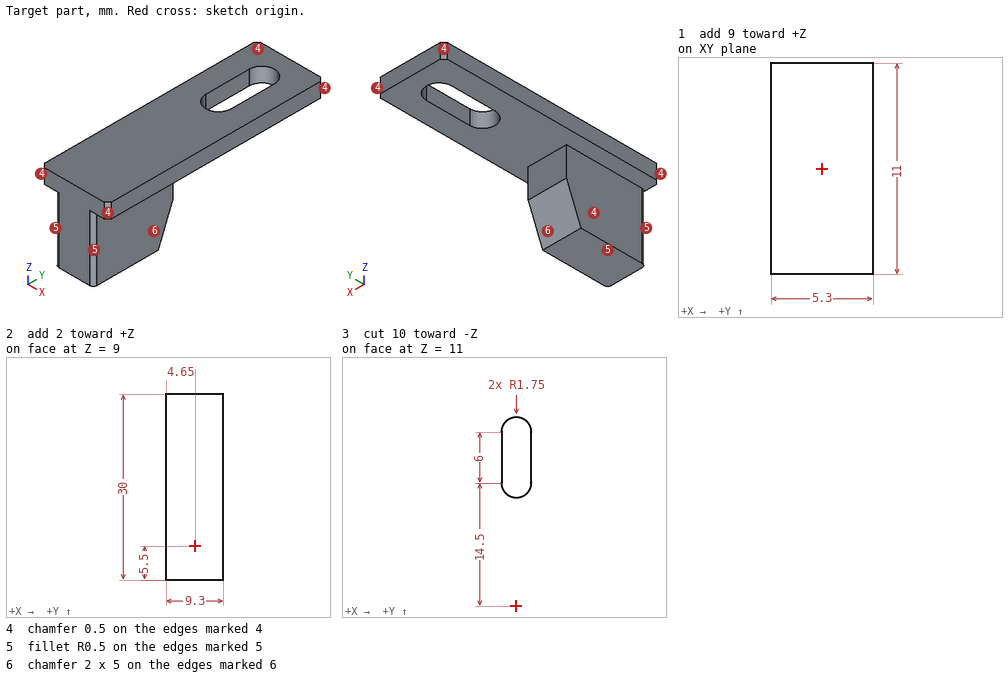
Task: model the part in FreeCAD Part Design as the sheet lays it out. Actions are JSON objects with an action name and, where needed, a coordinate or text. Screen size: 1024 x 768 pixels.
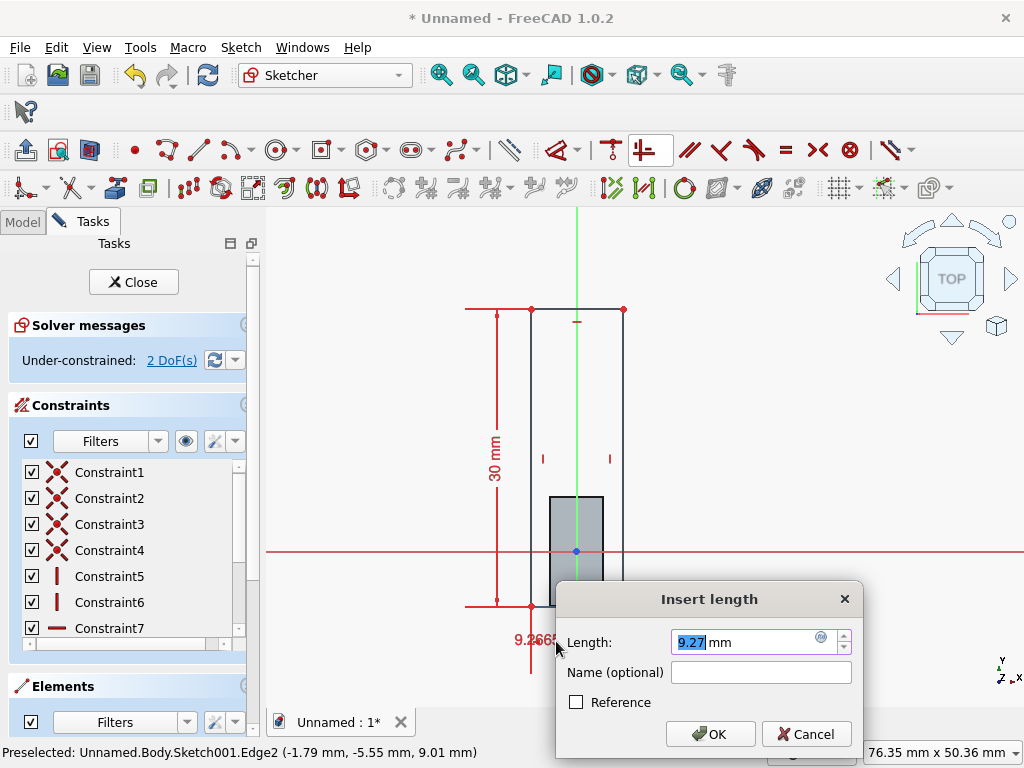
{"action": "type", "text": "9.3"}
{"action": "key", "text": "Return"}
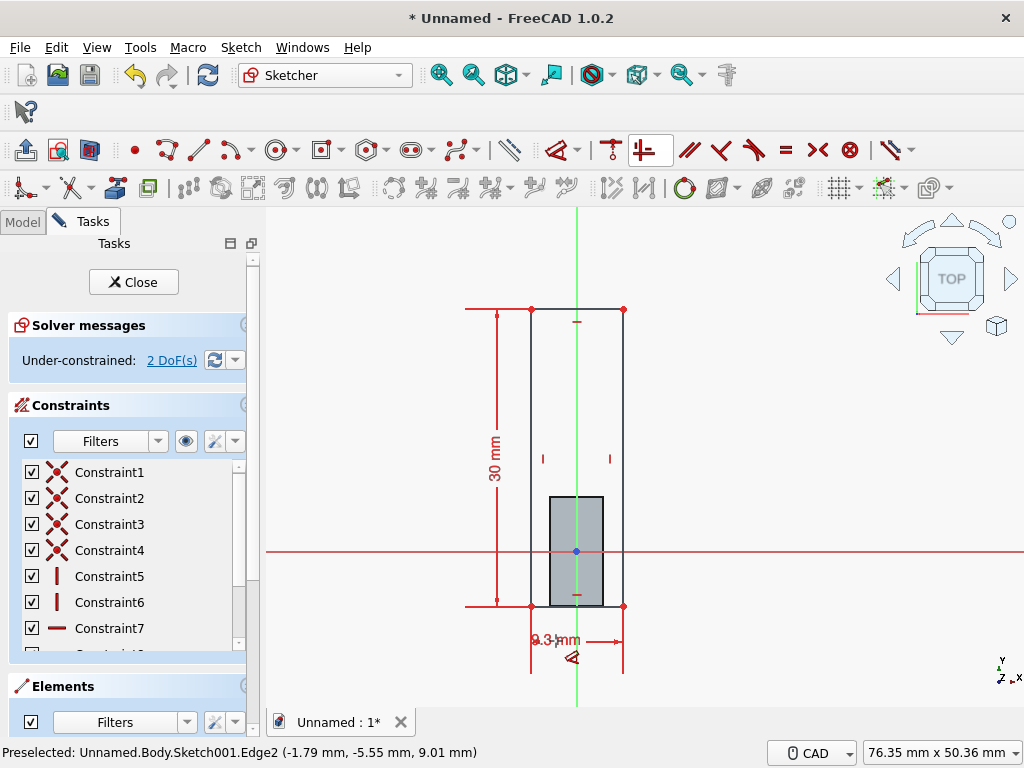
{"action": "left_click", "coordinate": [531, 607]}
{"action": "left_click", "coordinate": [497, 579]}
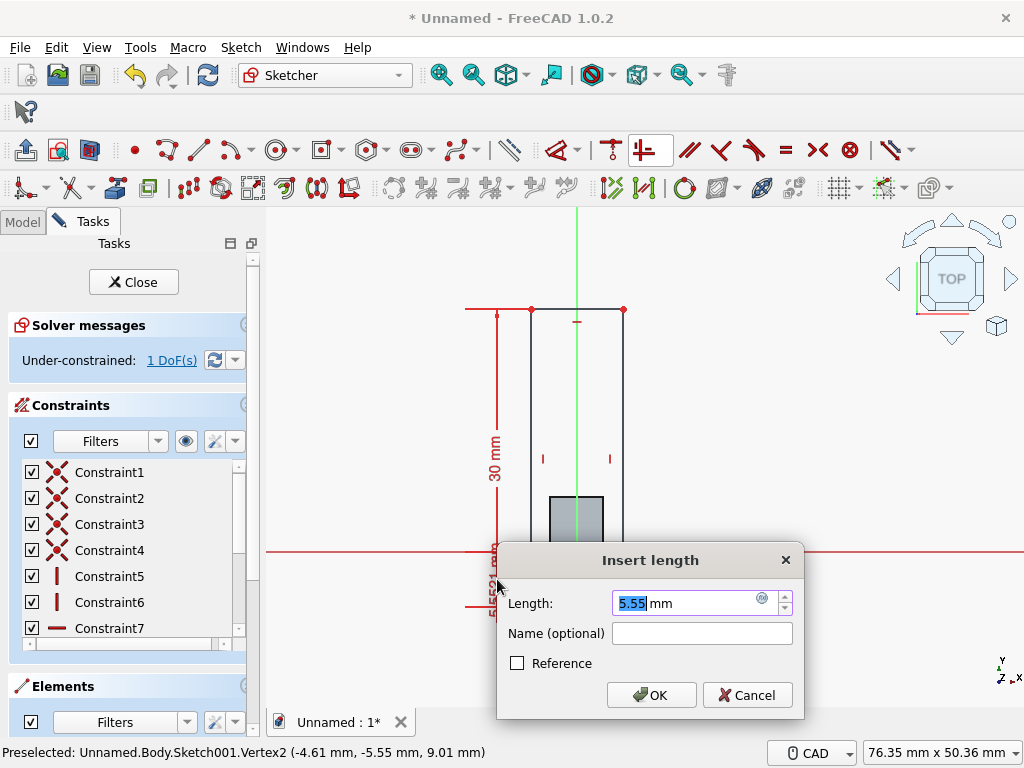
{"action": "type", "text": "5.5"}
{"action": "key", "text": "Return"}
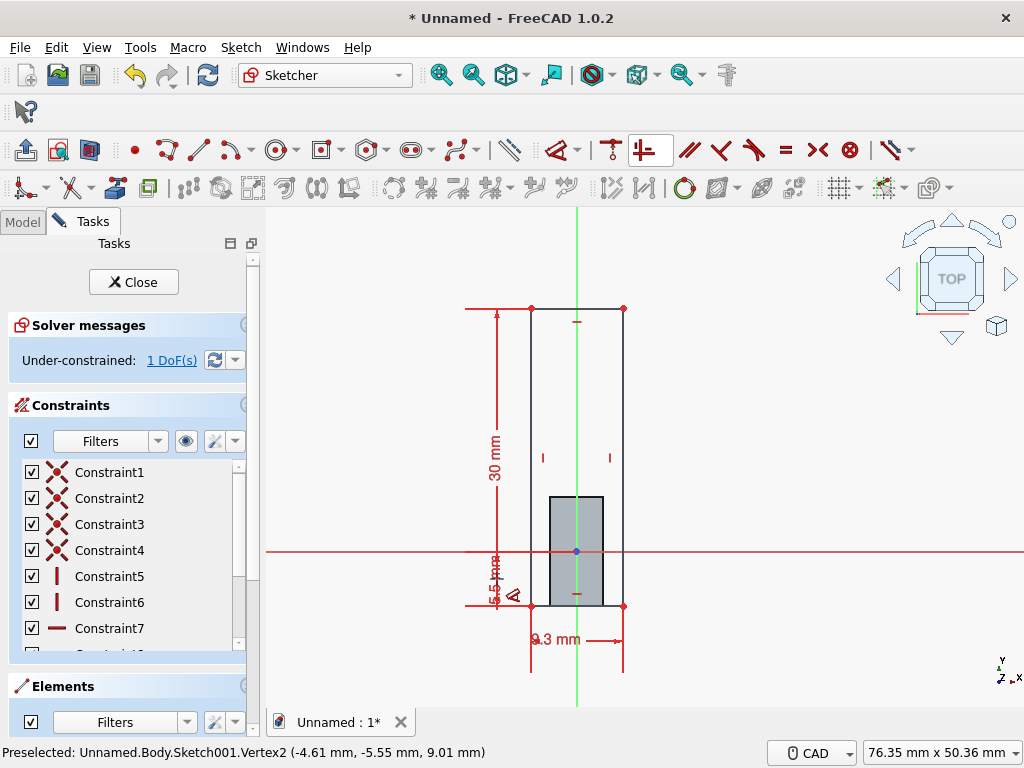
{"action": "left_click", "coordinate": [531, 309]}
{"action": "left_click", "coordinate": [554, 275]}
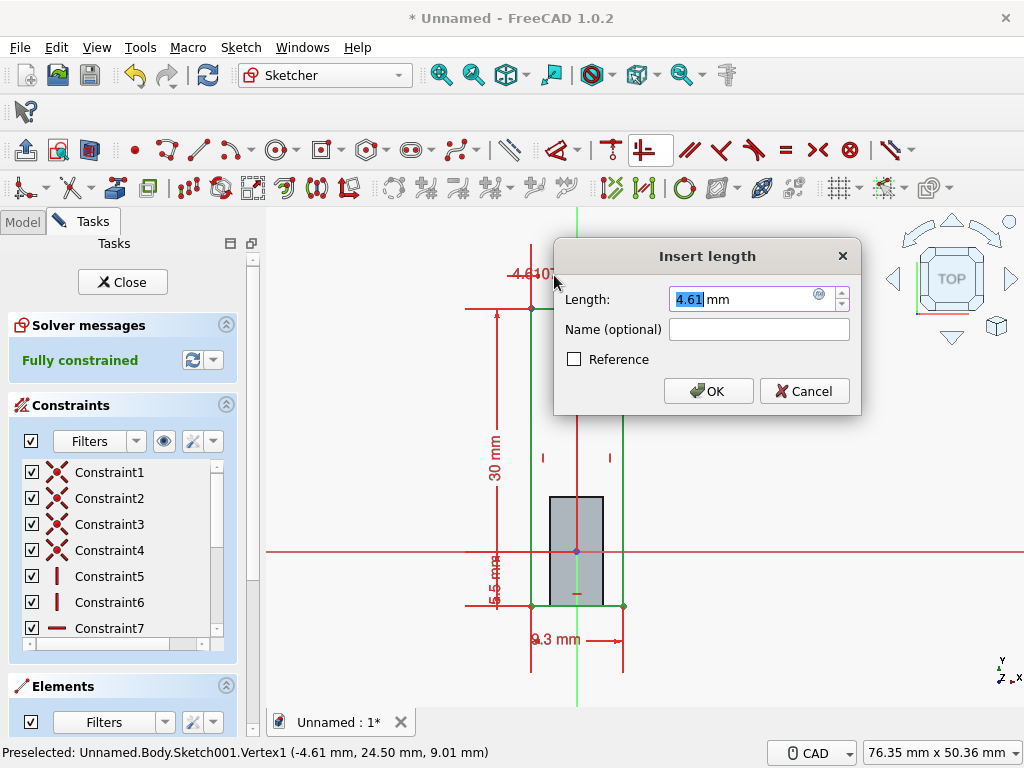
{"action": "type", "text": "4.65"}
{"action": "key", "text": "Return"}
{"action": "key", "text": "Escape"}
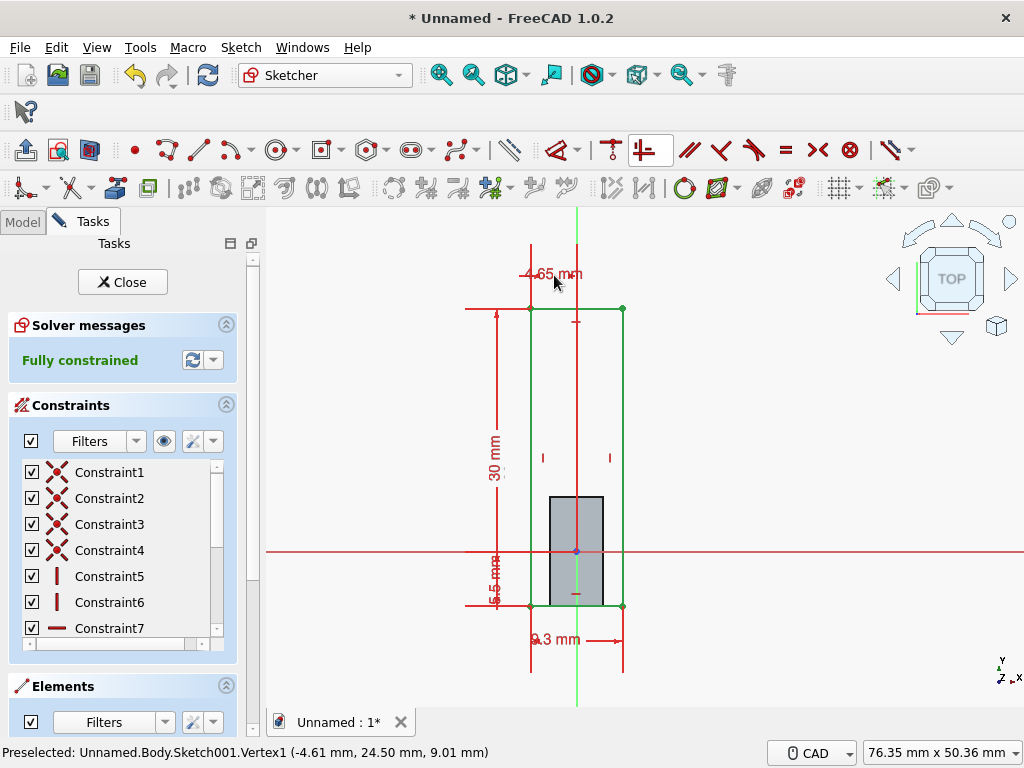
{"action": "left_click", "coordinate": [123, 282]}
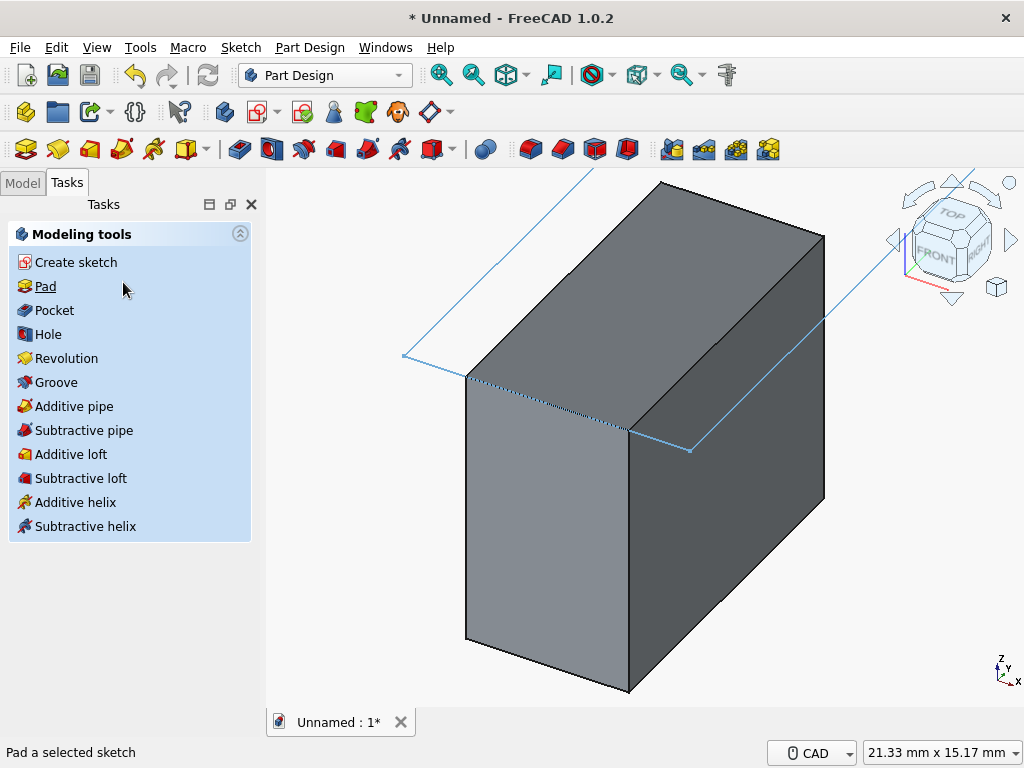
{"action": "left_click", "coordinate": [26, 150]}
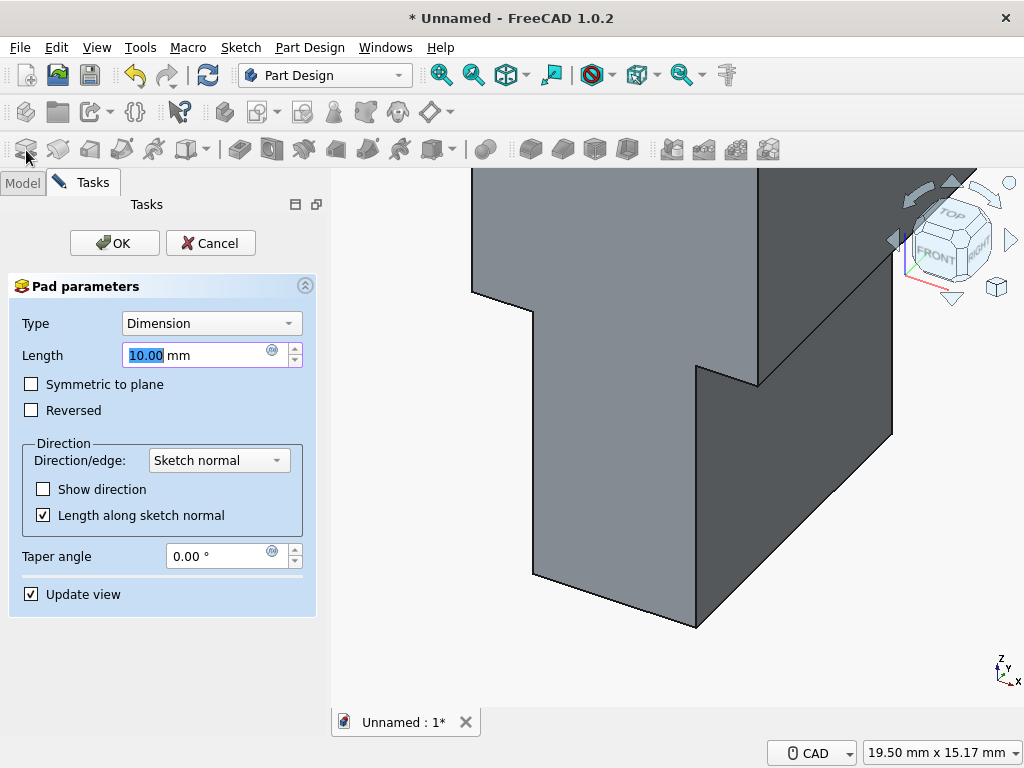
{"action": "type", "text": "2"}
{"action": "key", "text": "Tab"}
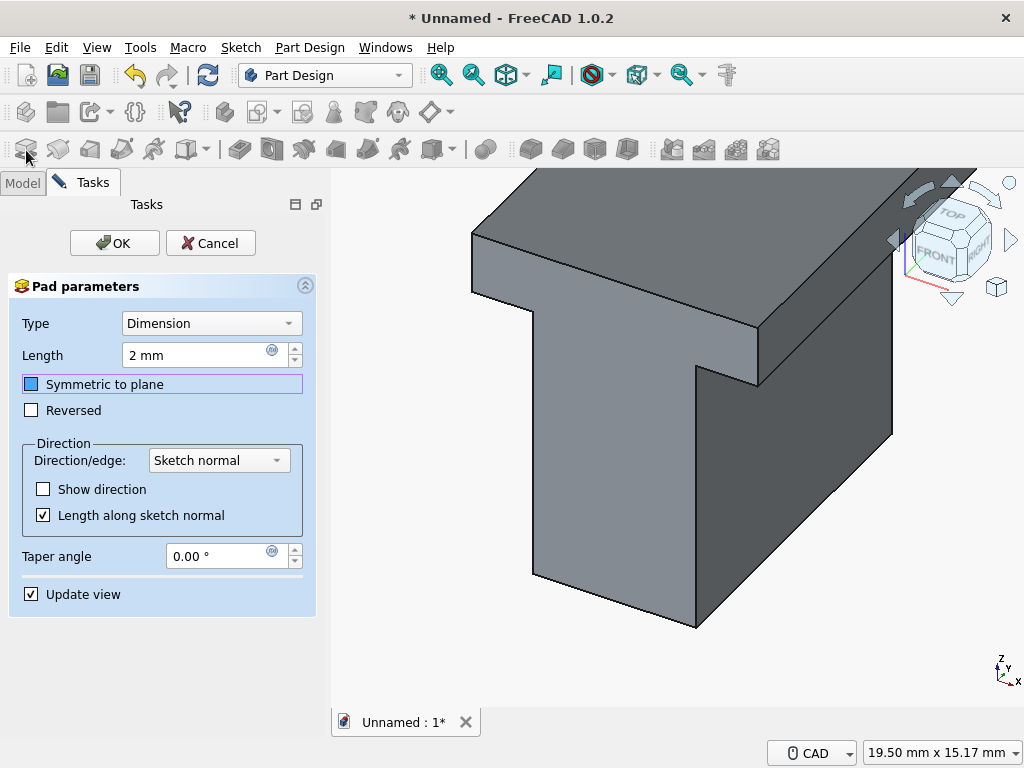
{"action": "left_click", "coordinate": [115, 243]}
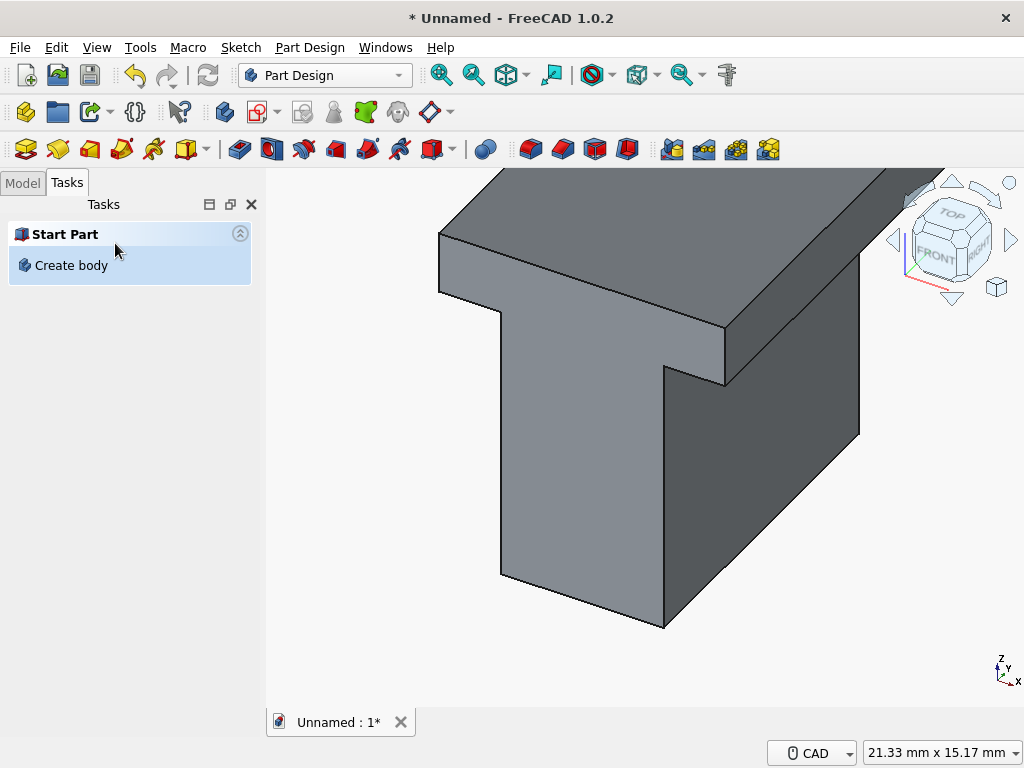
{"action": "left_click", "coordinate": [442, 76]}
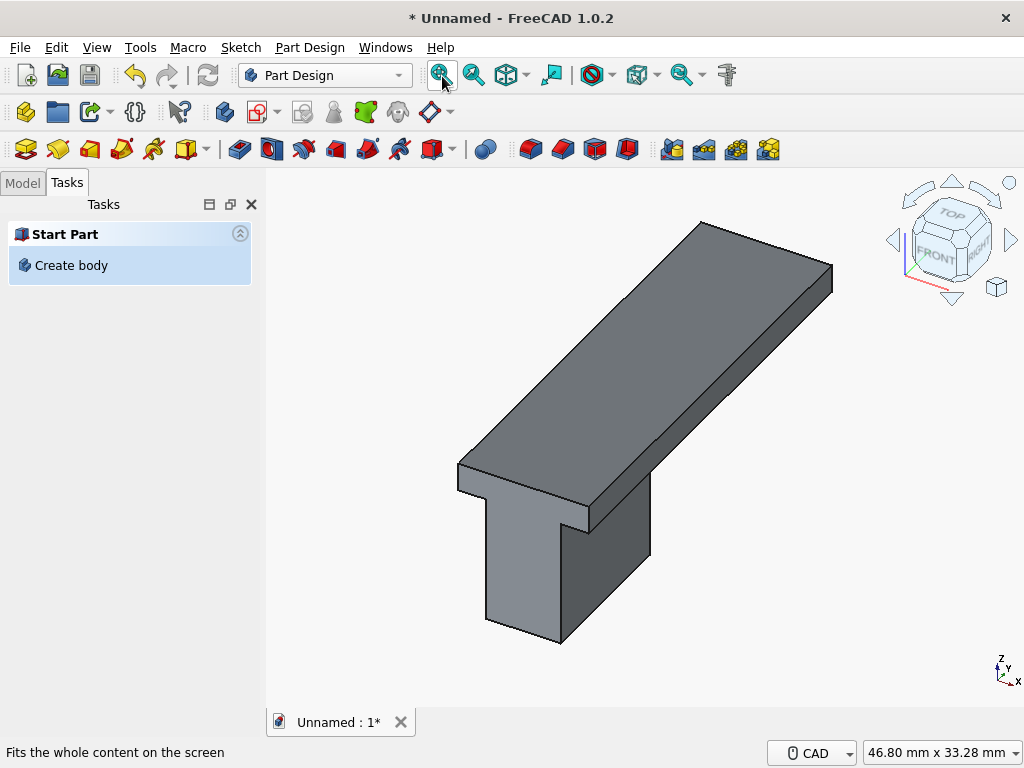
{"action": "left_click", "coordinate": [714, 295]}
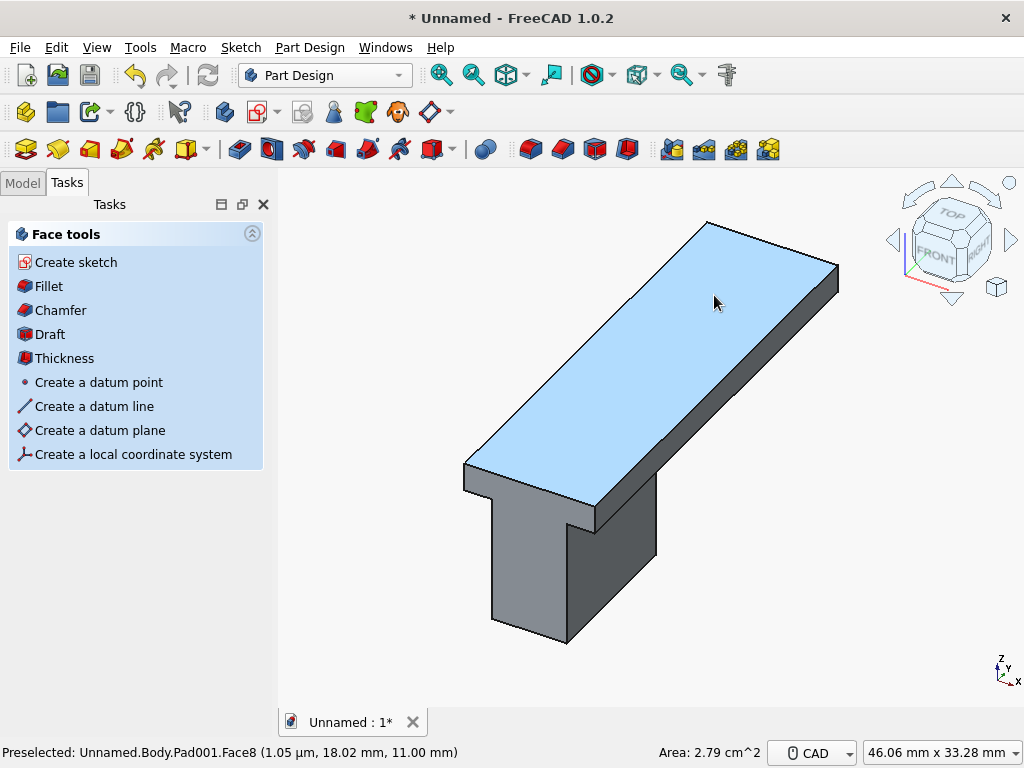
{"action": "left_click", "coordinate": [258, 112]}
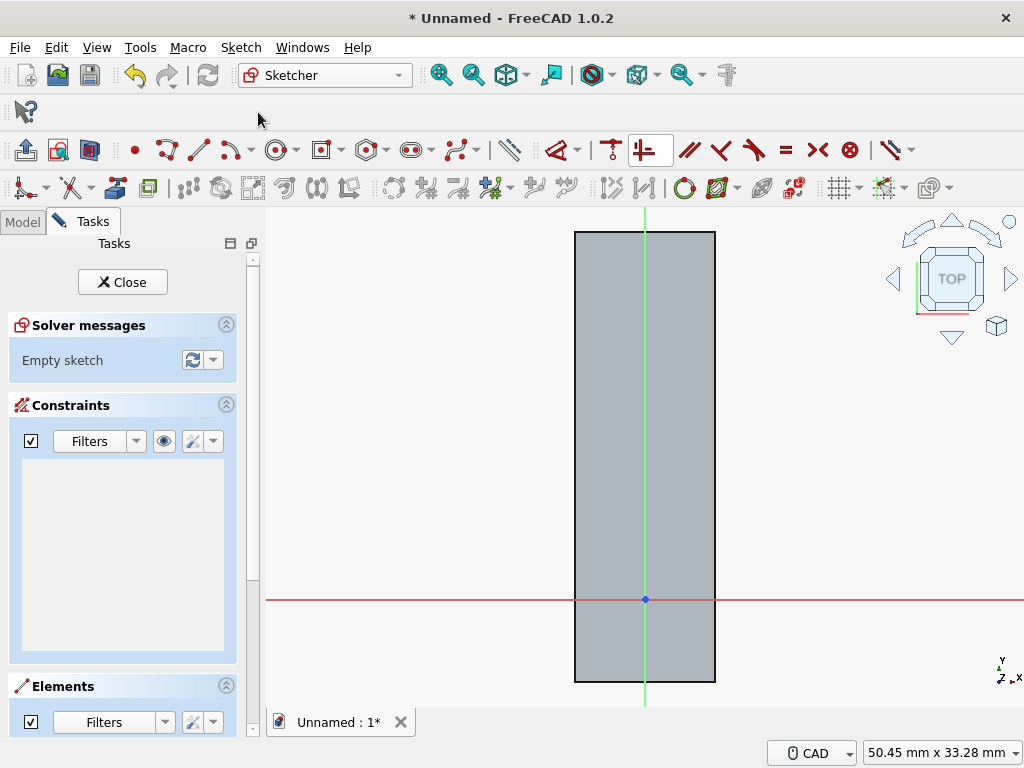
{"action": "key", "text": "g s"}